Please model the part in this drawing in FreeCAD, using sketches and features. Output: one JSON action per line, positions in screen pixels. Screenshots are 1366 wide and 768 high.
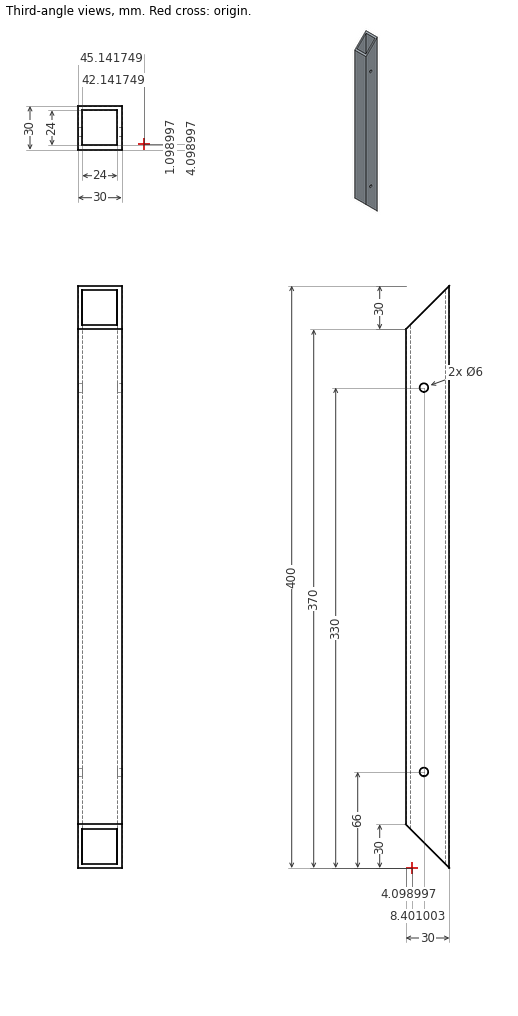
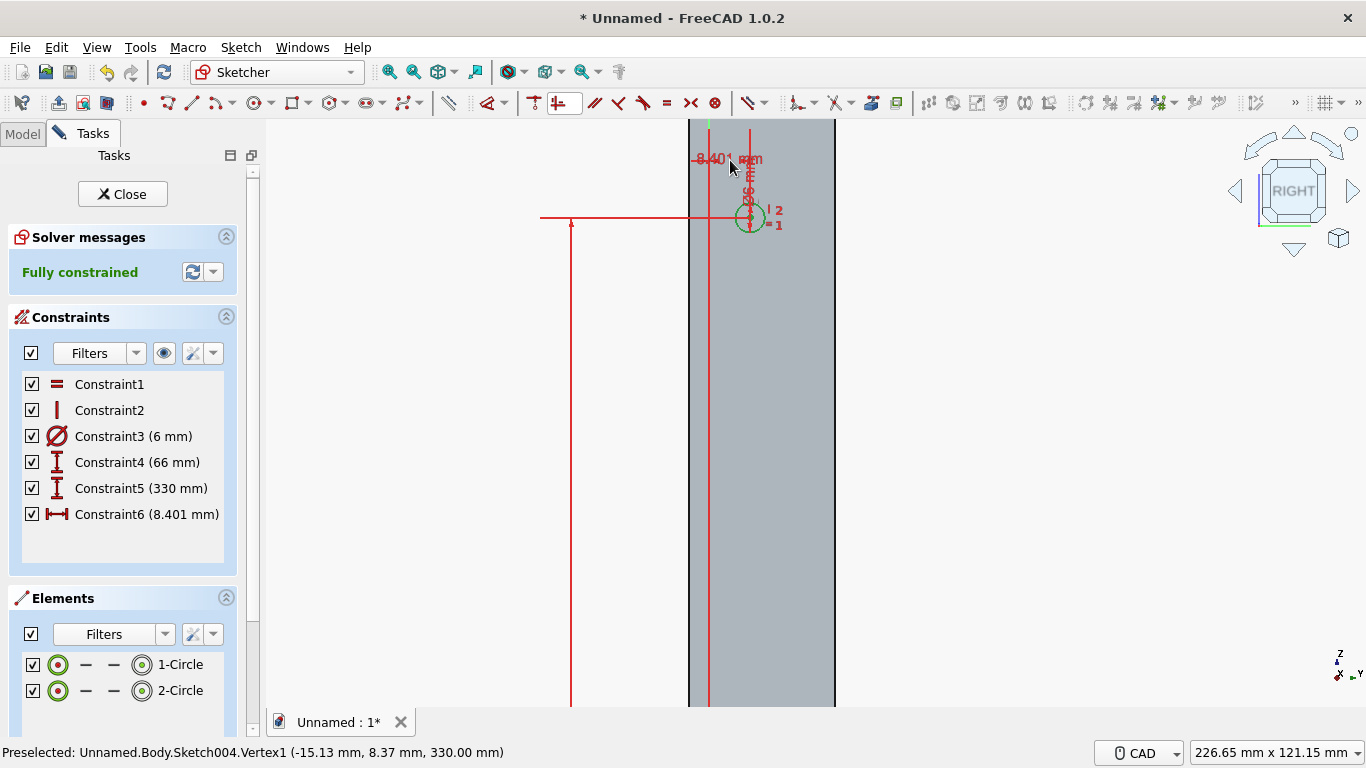
{"action": "left_click", "coordinate": [123, 194]}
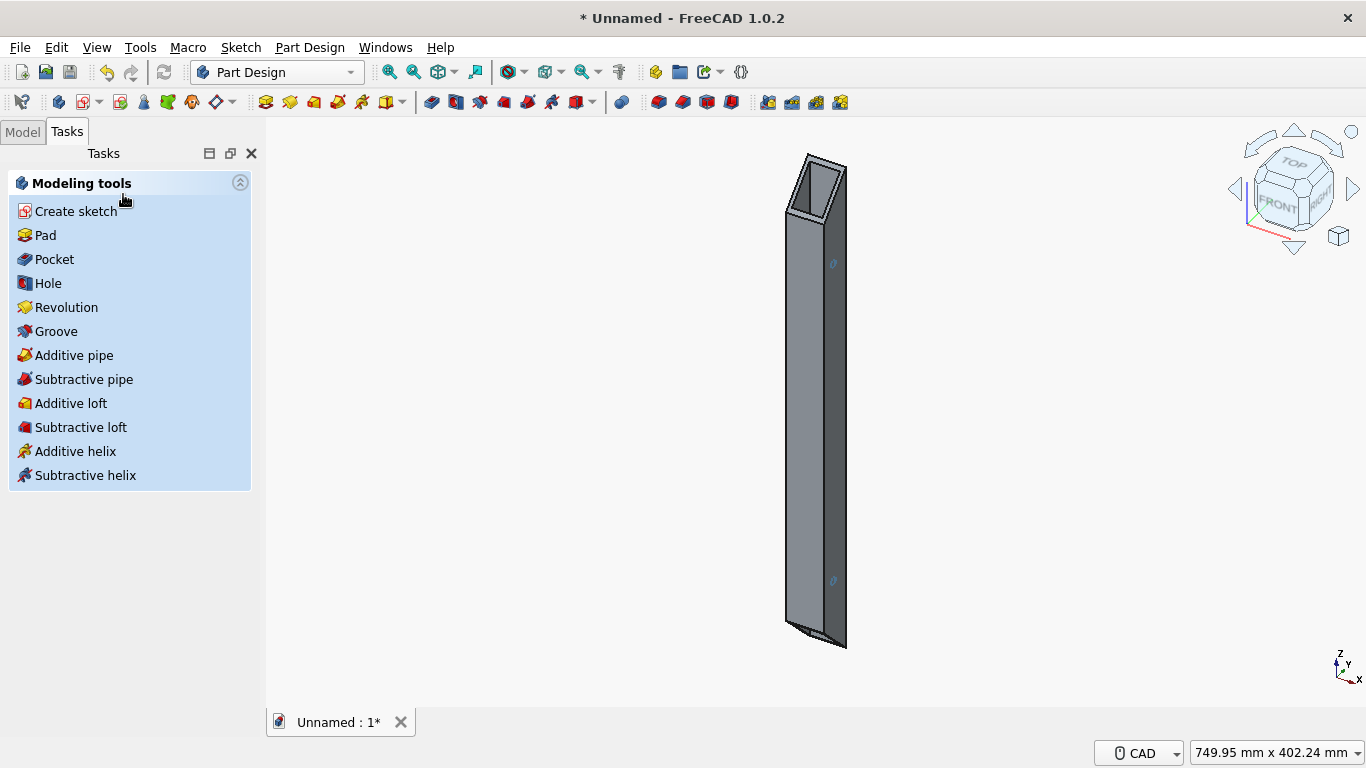
{"action": "left_click", "coordinate": [432, 102]}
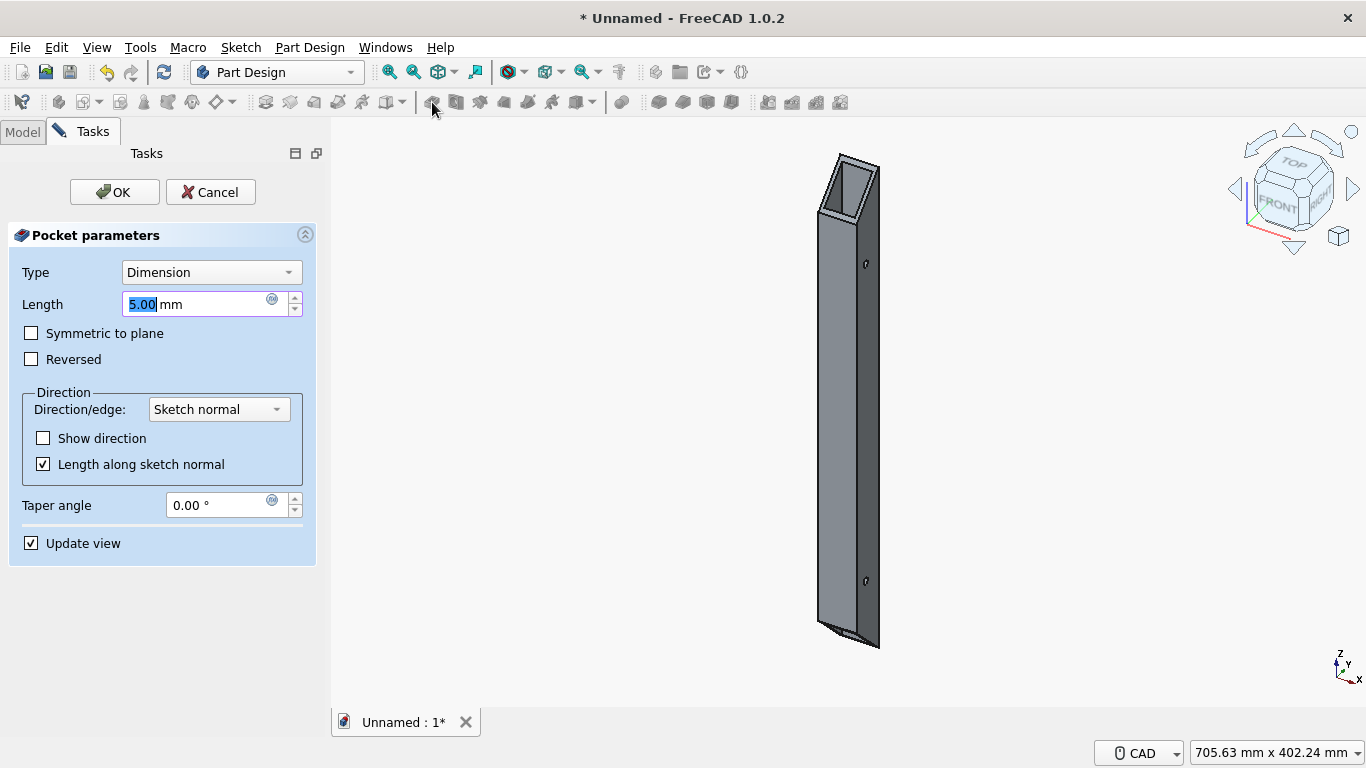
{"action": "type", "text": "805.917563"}
{"action": "key", "text": "Tab"}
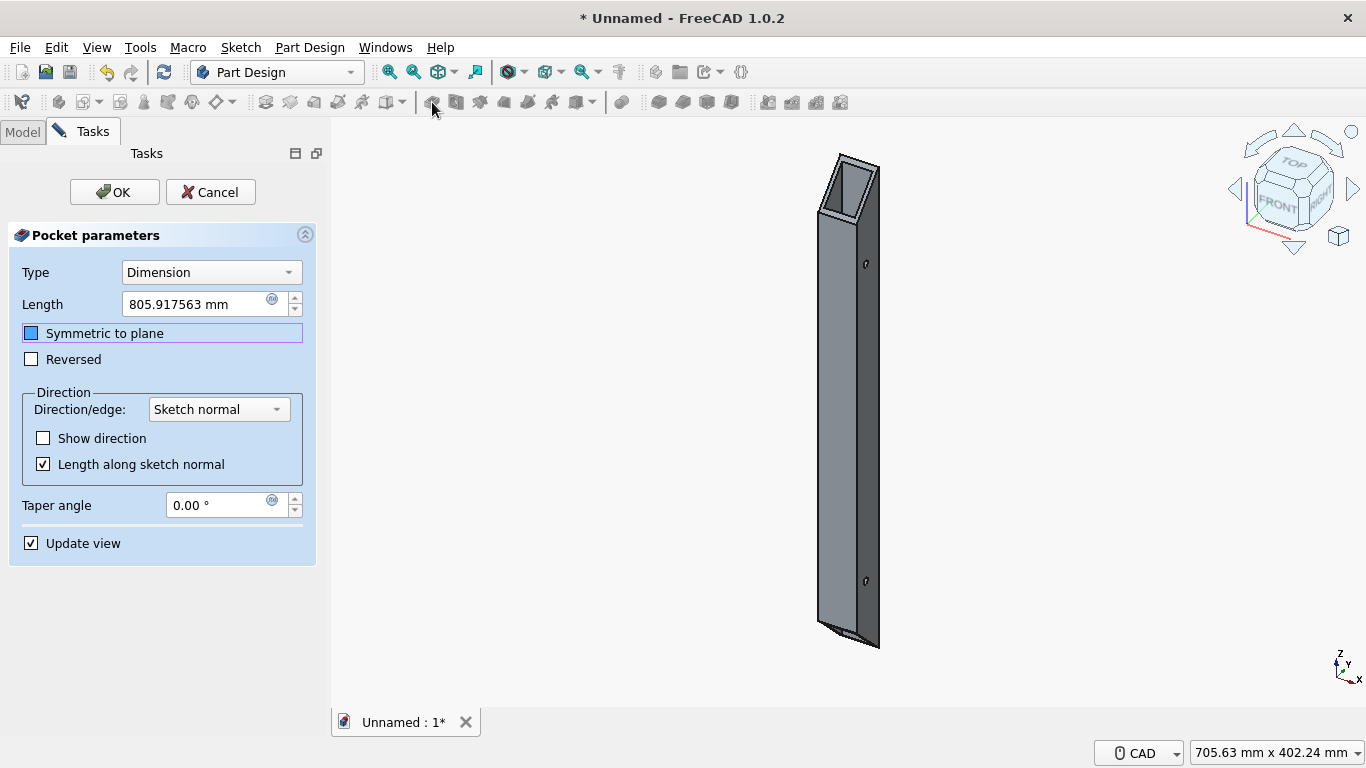
{"action": "left_click", "coordinate": [30, 333]}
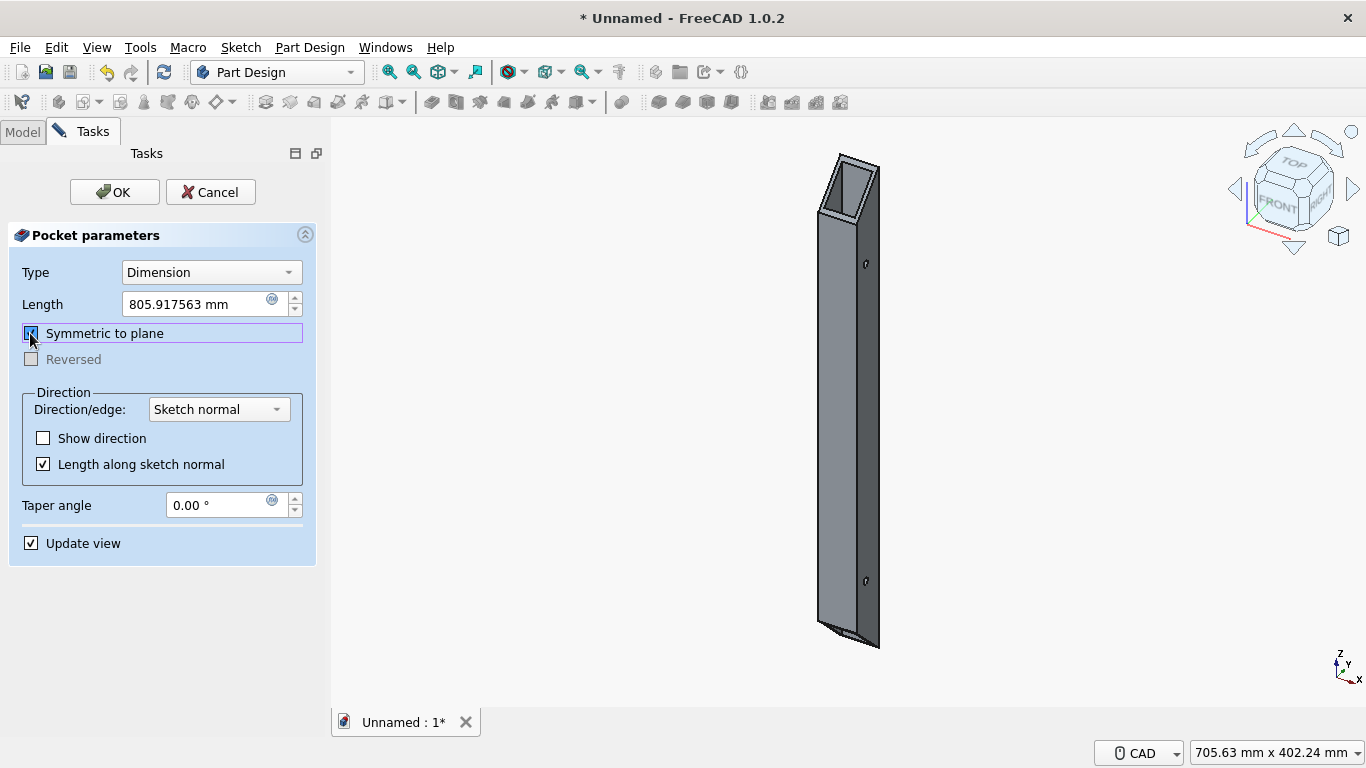
{"action": "left_click", "coordinate": [115, 192]}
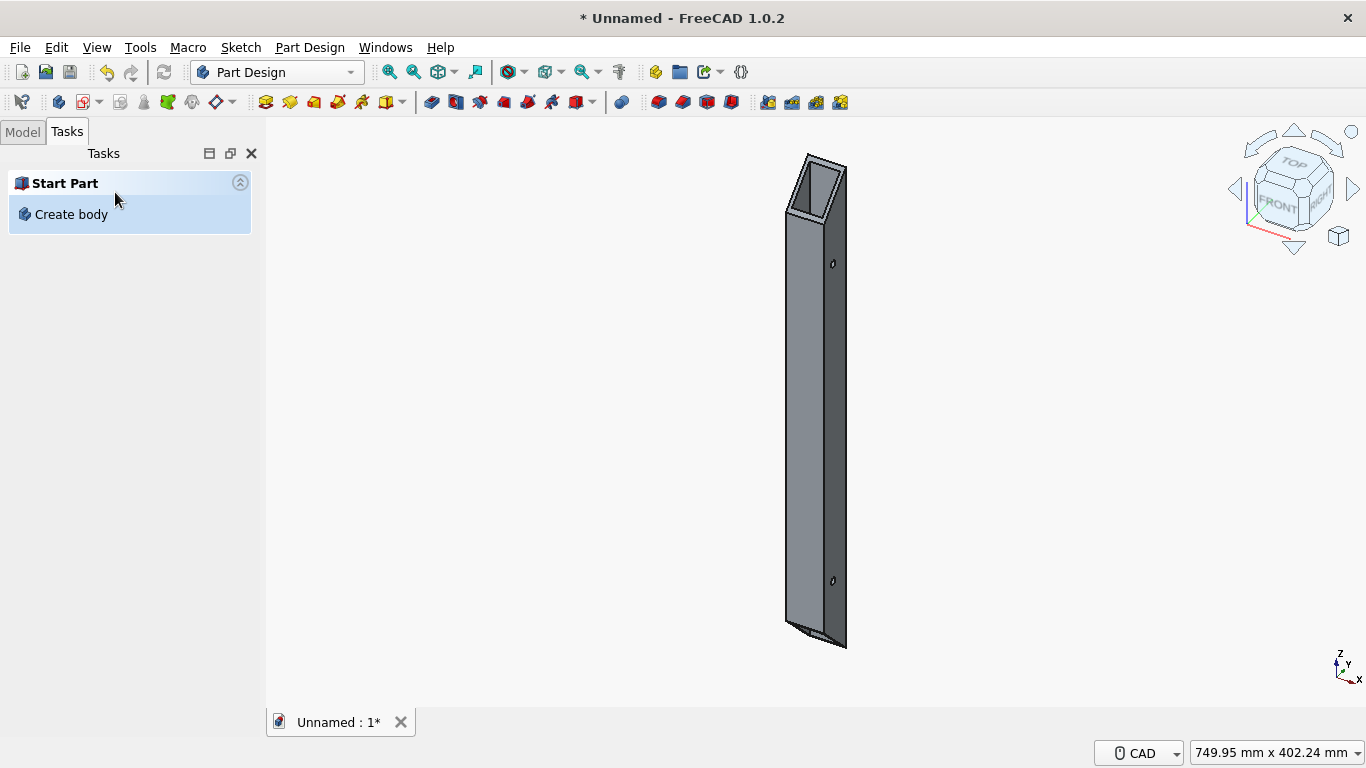
{"action": "key", "text": "0"}